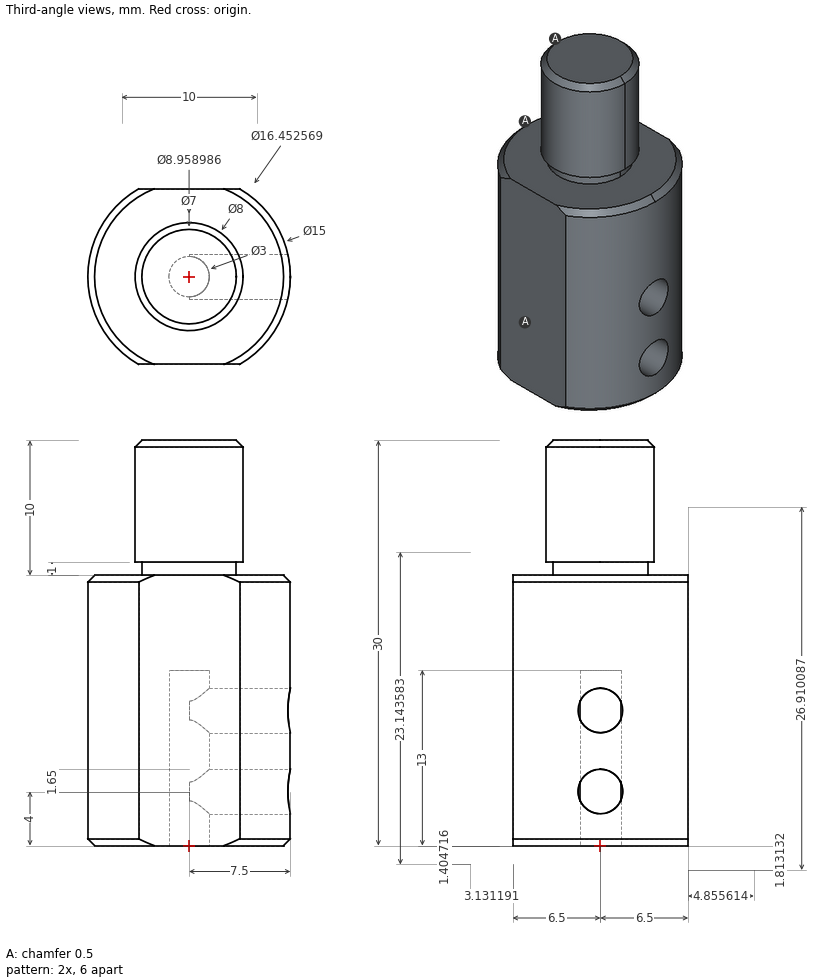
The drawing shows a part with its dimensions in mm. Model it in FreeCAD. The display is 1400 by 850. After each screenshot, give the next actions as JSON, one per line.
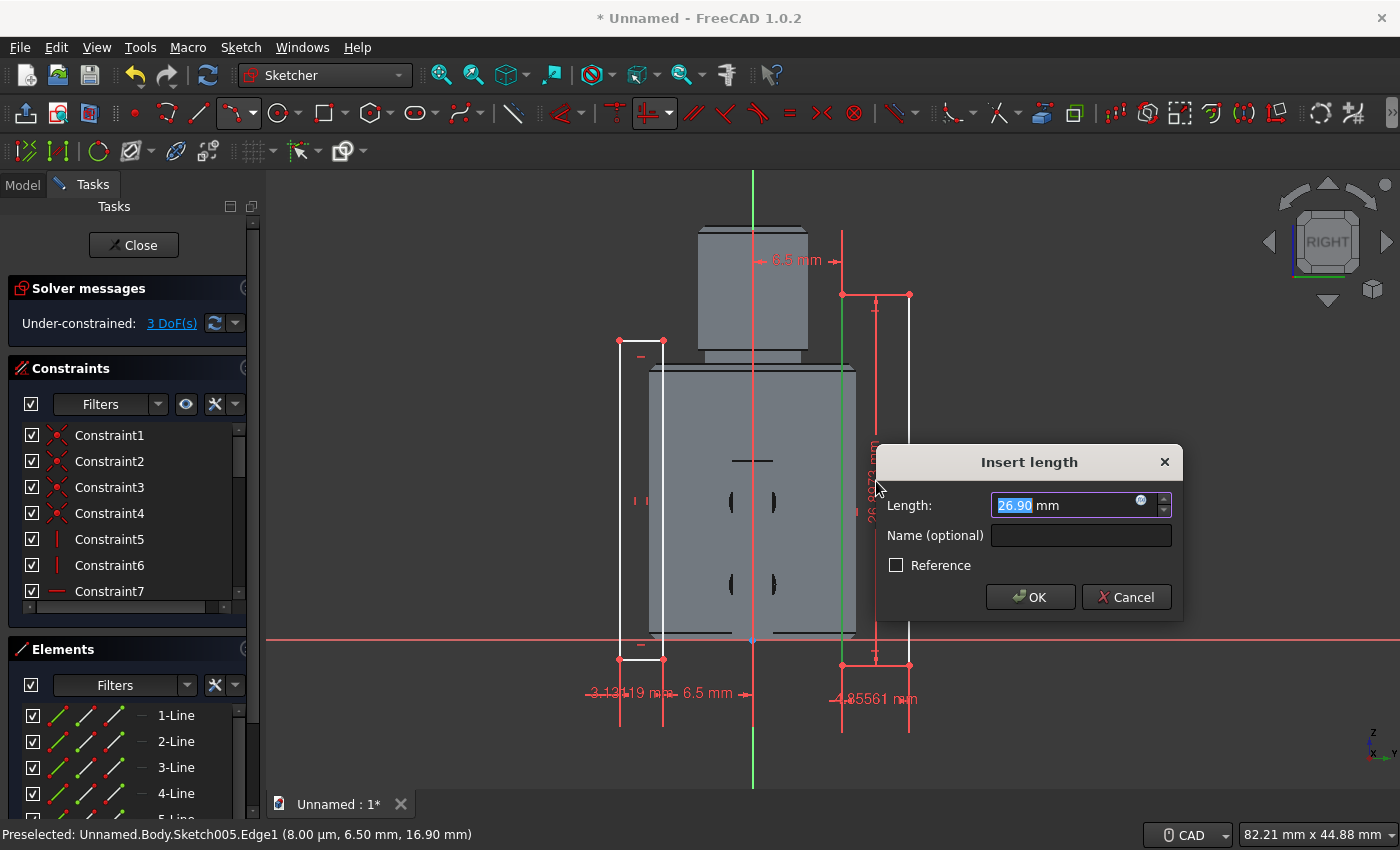
{"action": "type", "text": "26.910087"}
{"action": "key", "text": "Return"}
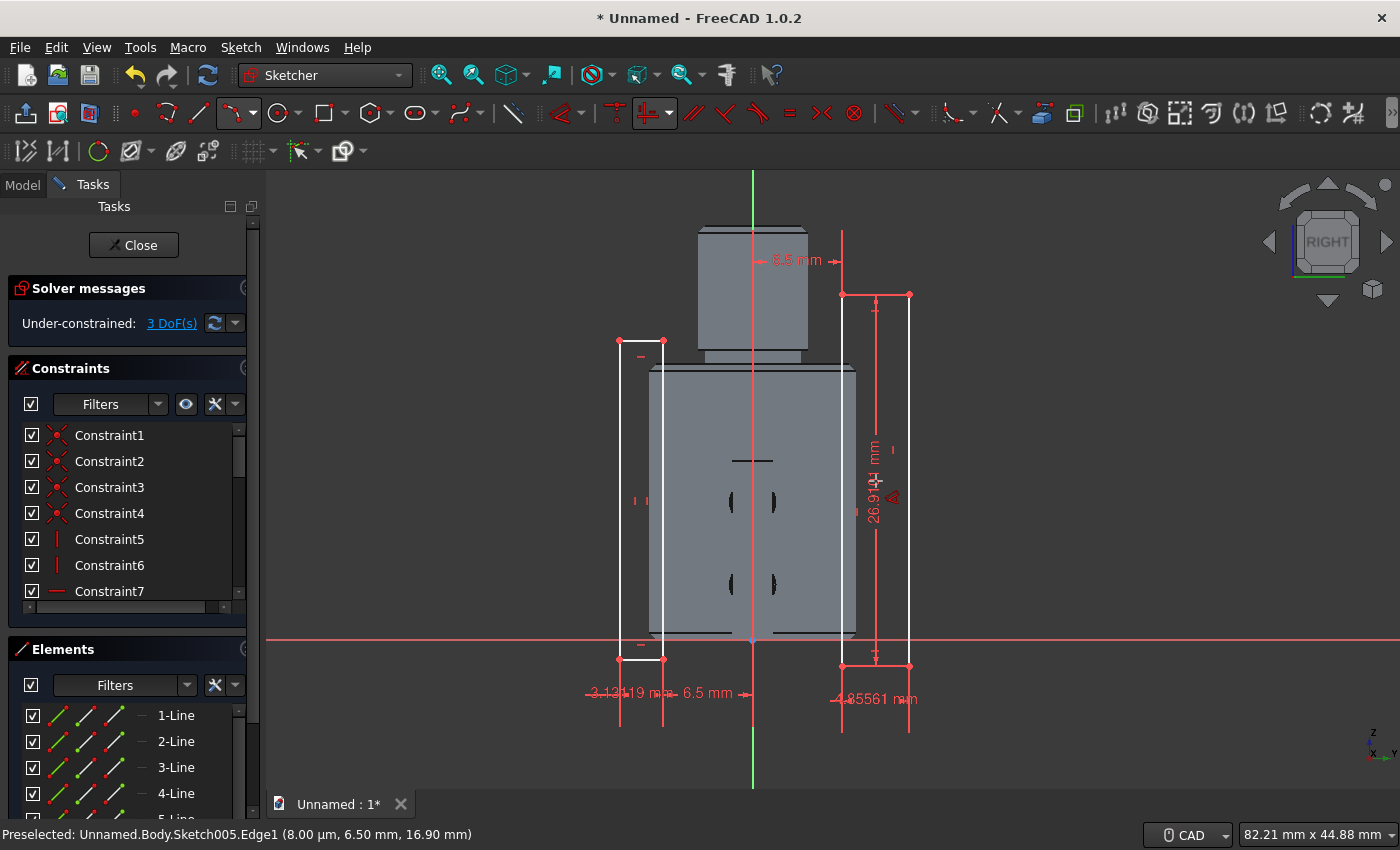
{"action": "left_click", "coordinate": [620, 437]}
{"action": "left_click", "coordinate": [586, 501]}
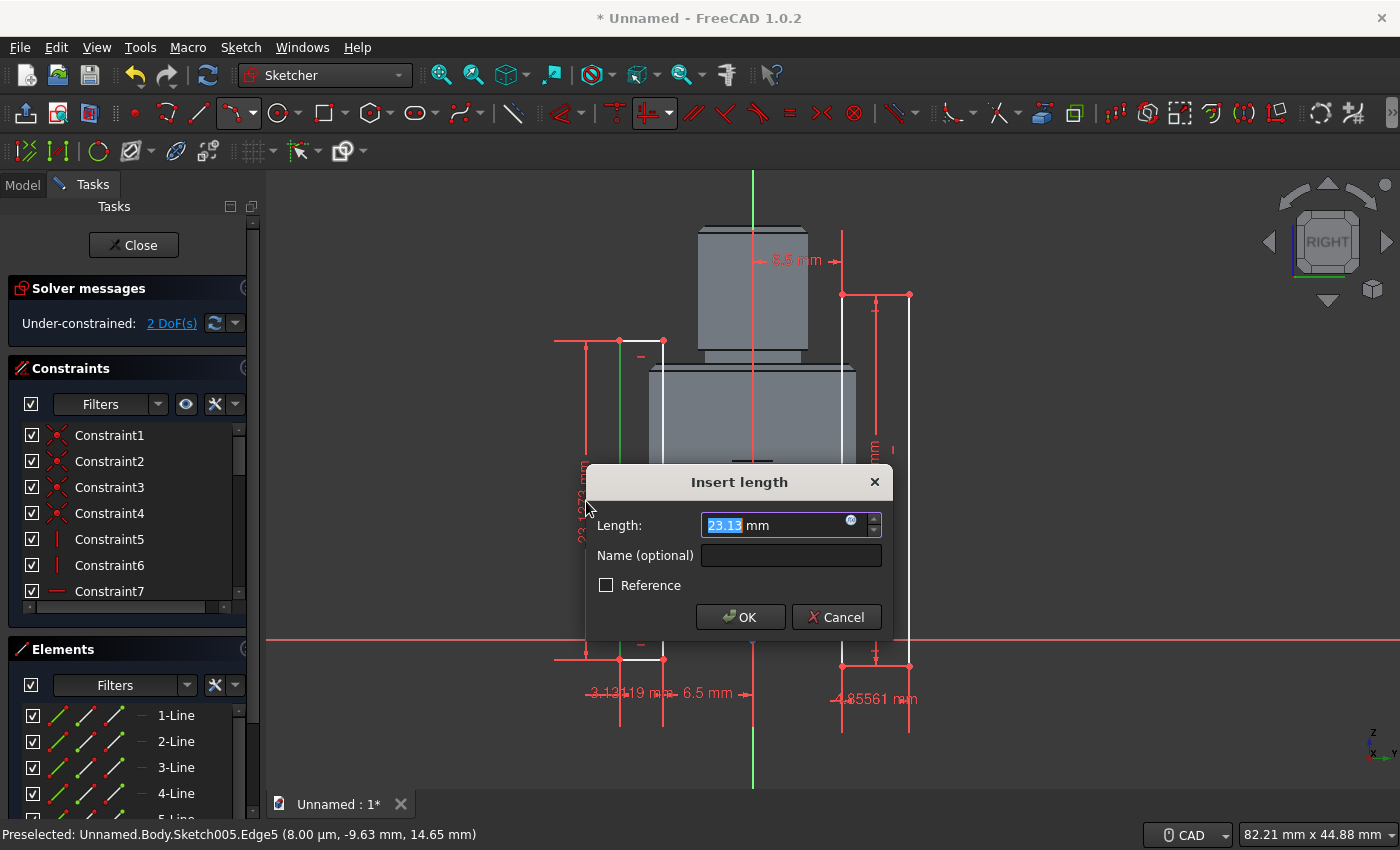
{"action": "type", "text": "23.143583"}
{"action": "key", "text": "Return"}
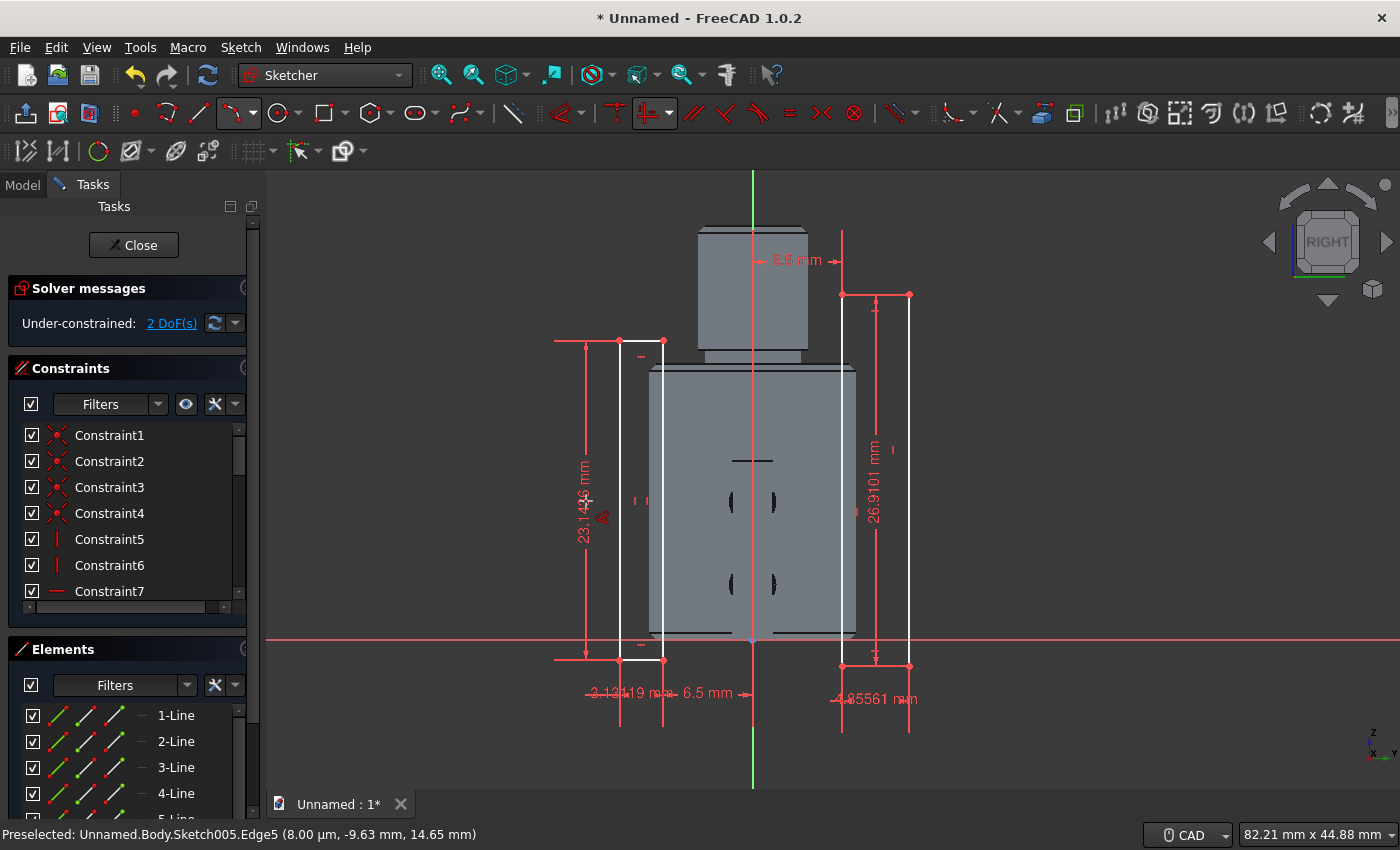
{"action": "scroll", "coordinate": [842, 666], "scroll_direction": "up", "scroll_amount": 3}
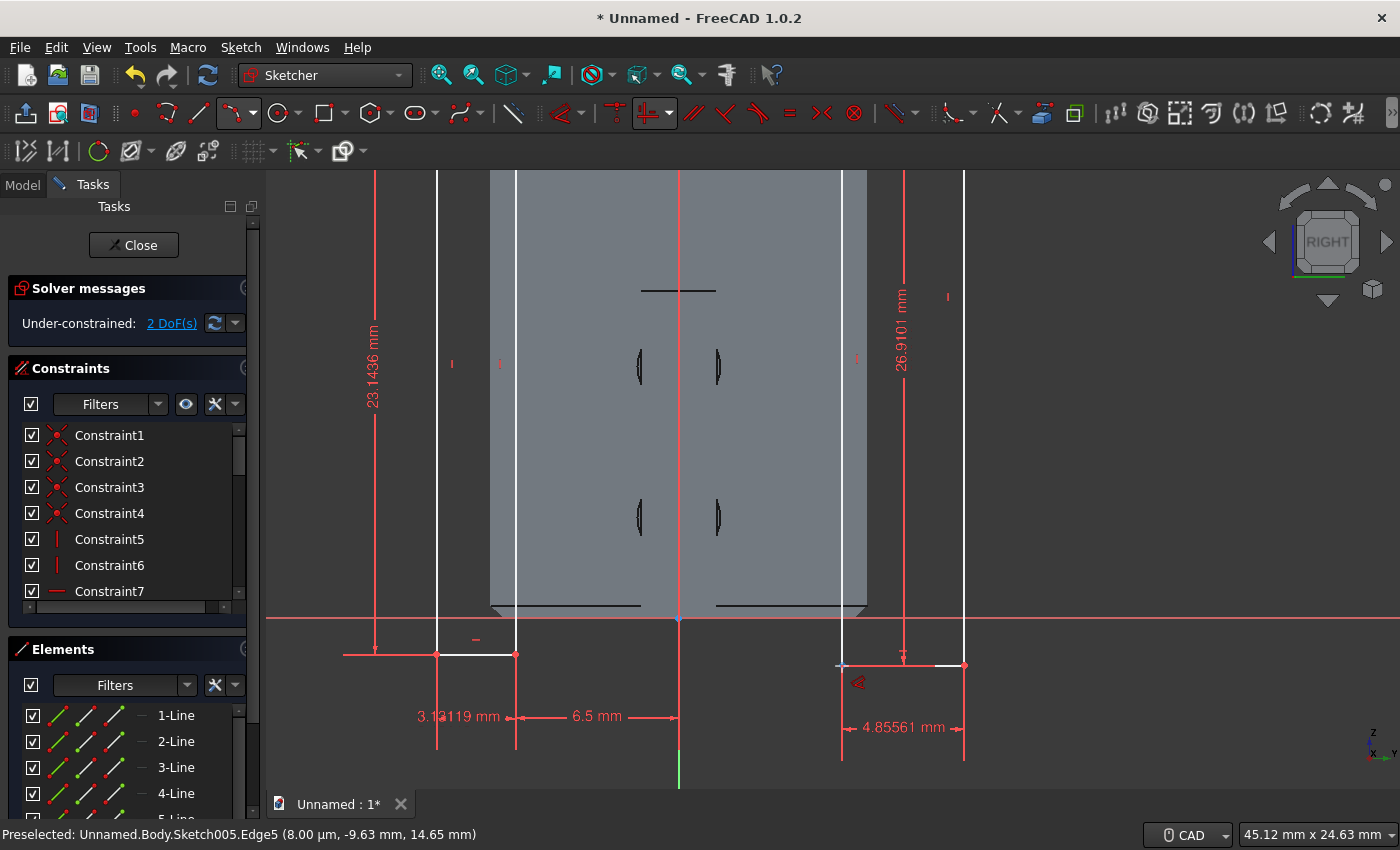
{"action": "left_click", "coordinate": [842, 666]}
{"action": "left_click", "coordinate": [876, 642]}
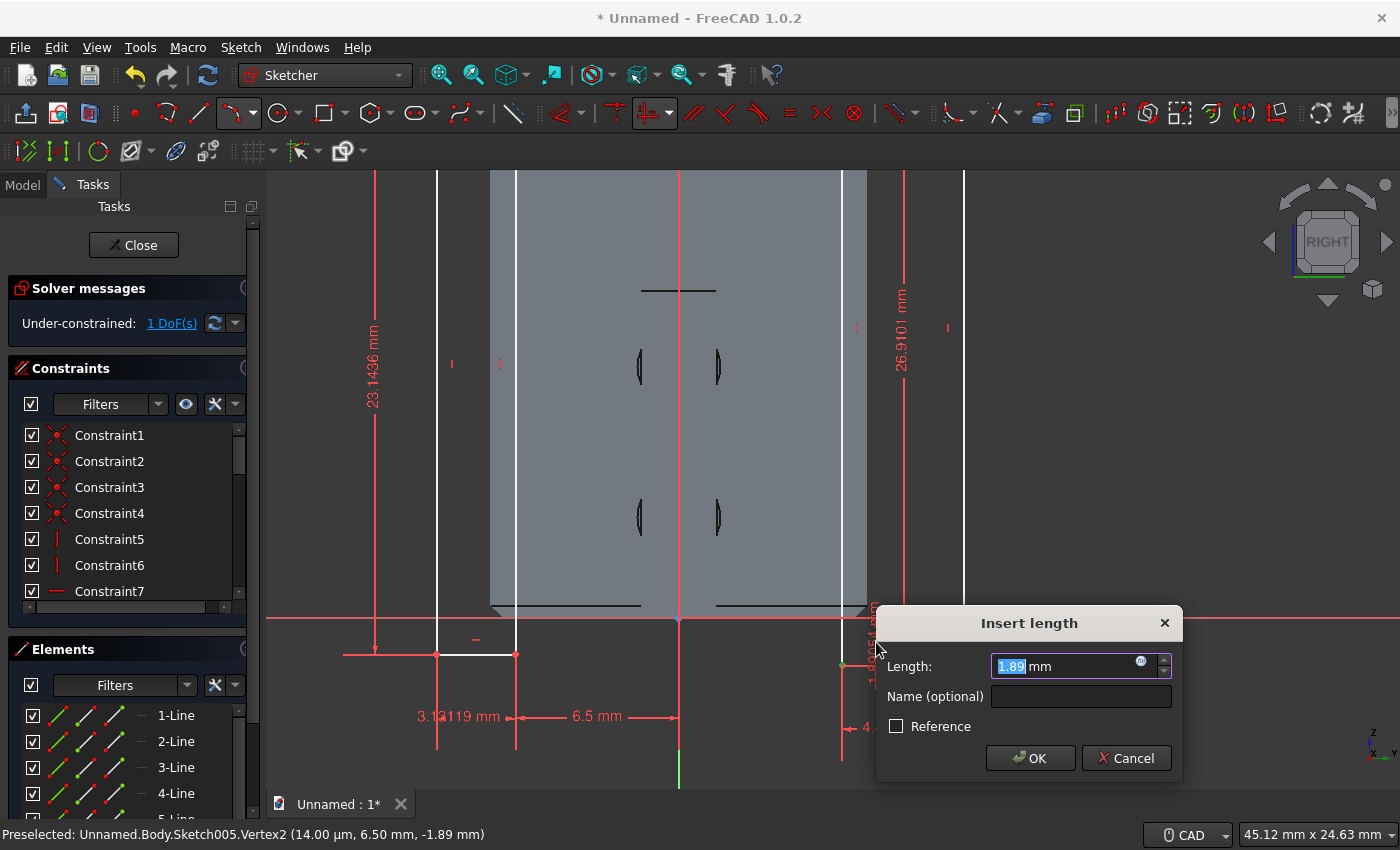
{"action": "type", "text": "1.813132"}
{"action": "key", "text": "Return"}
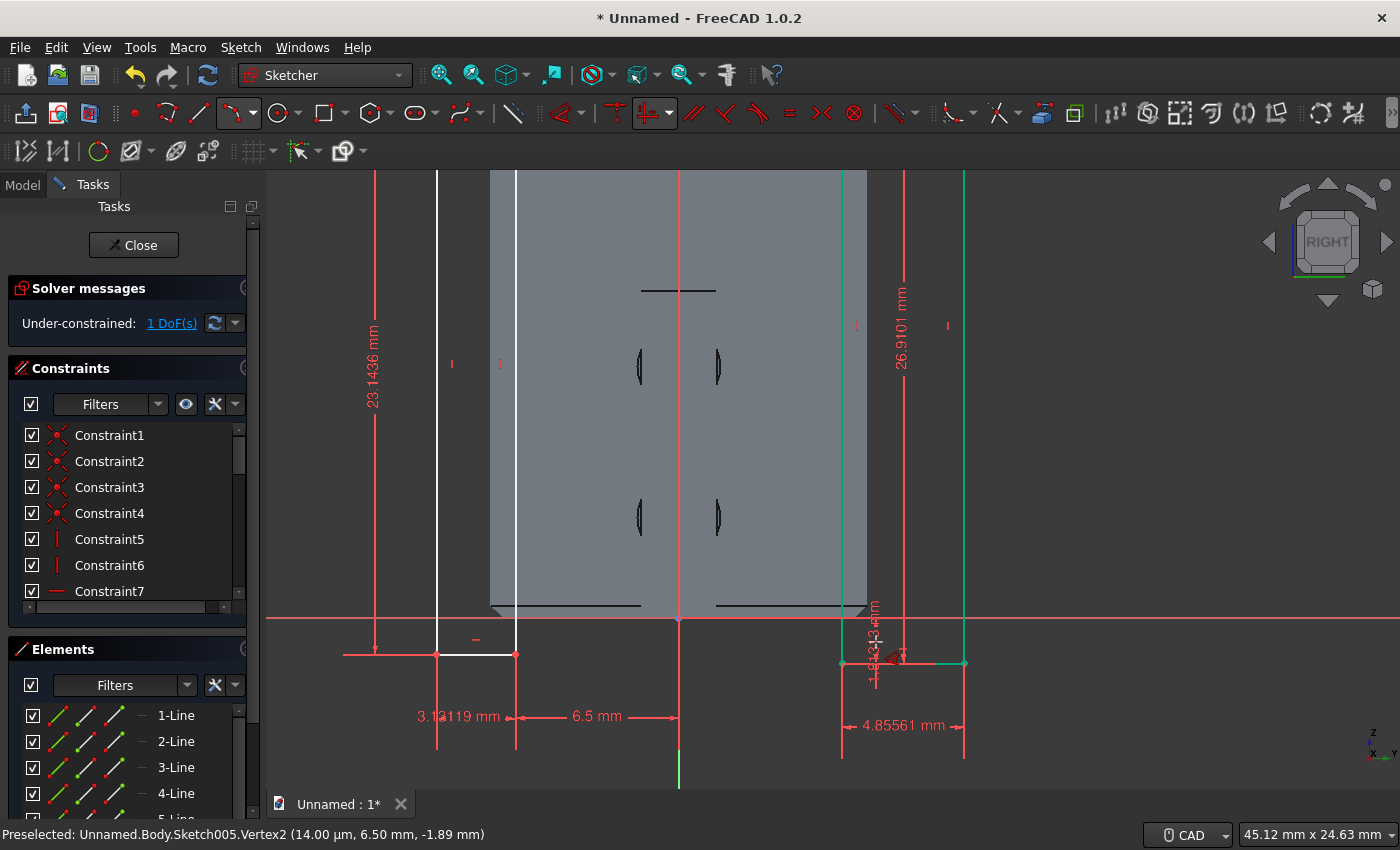
{"action": "left_click", "coordinate": [437, 655]}
{"action": "left_click", "coordinate": [403, 636]}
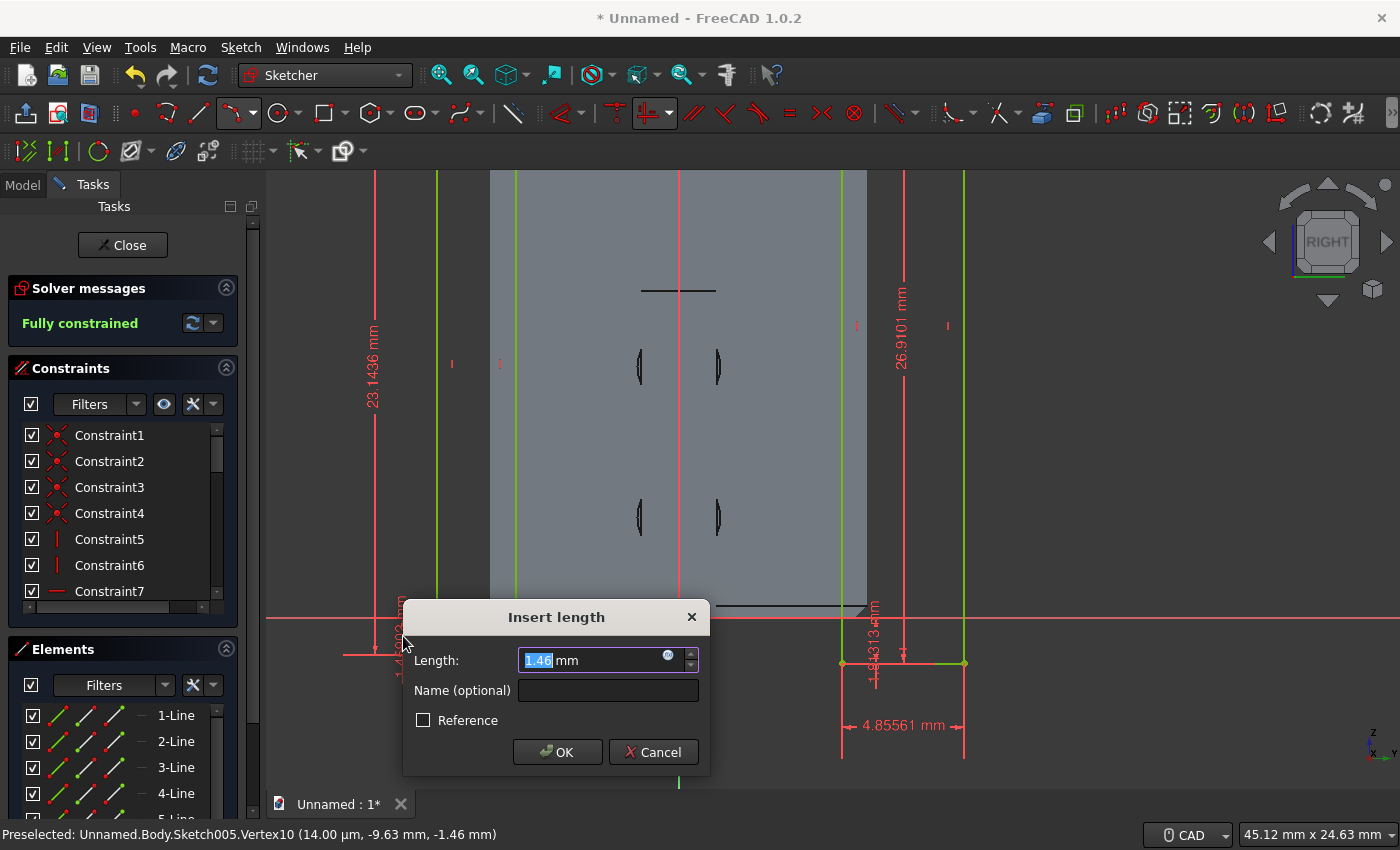
{"action": "type", "text": "1.404716"}
{"action": "key", "text": "Return"}
{"action": "key", "text": "Escape"}